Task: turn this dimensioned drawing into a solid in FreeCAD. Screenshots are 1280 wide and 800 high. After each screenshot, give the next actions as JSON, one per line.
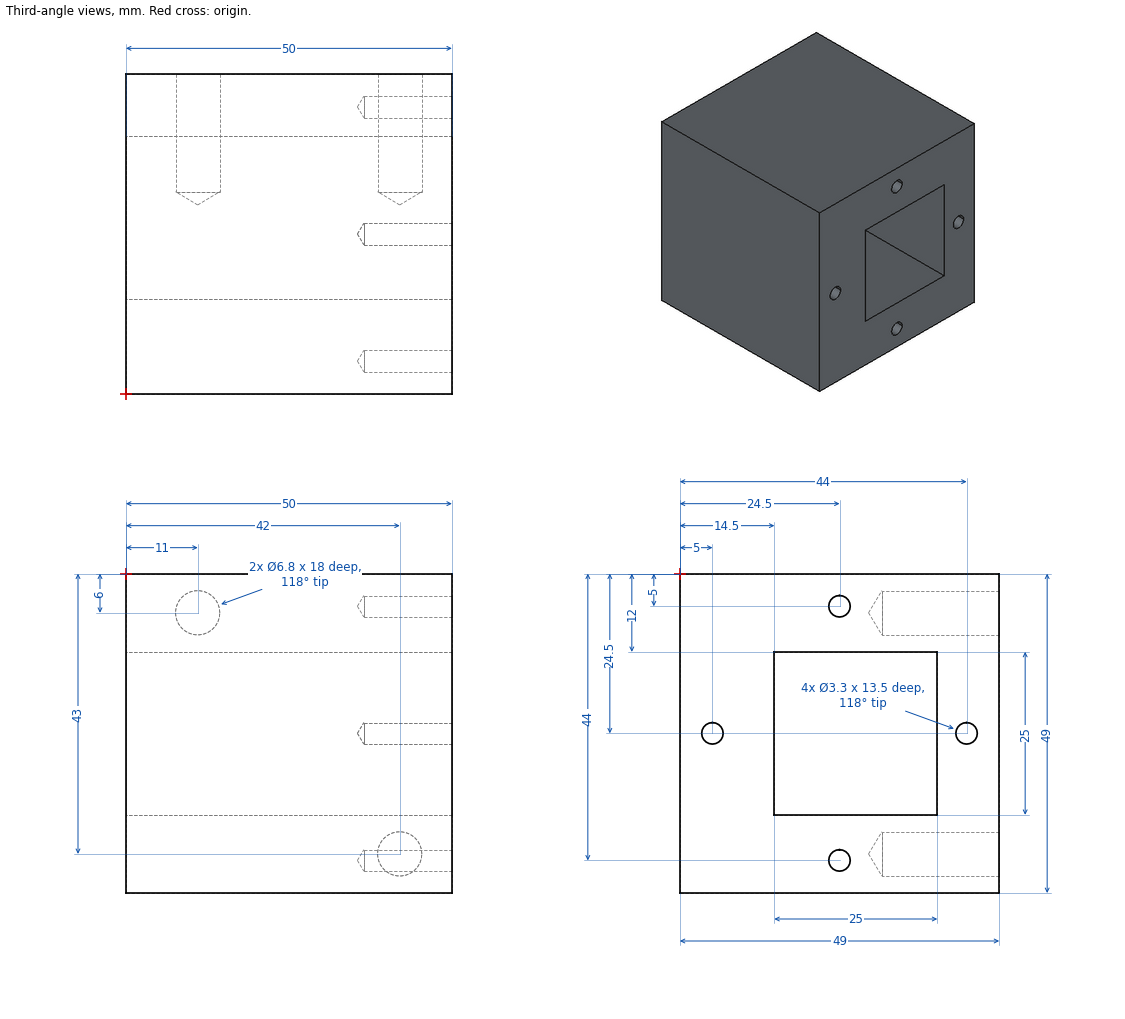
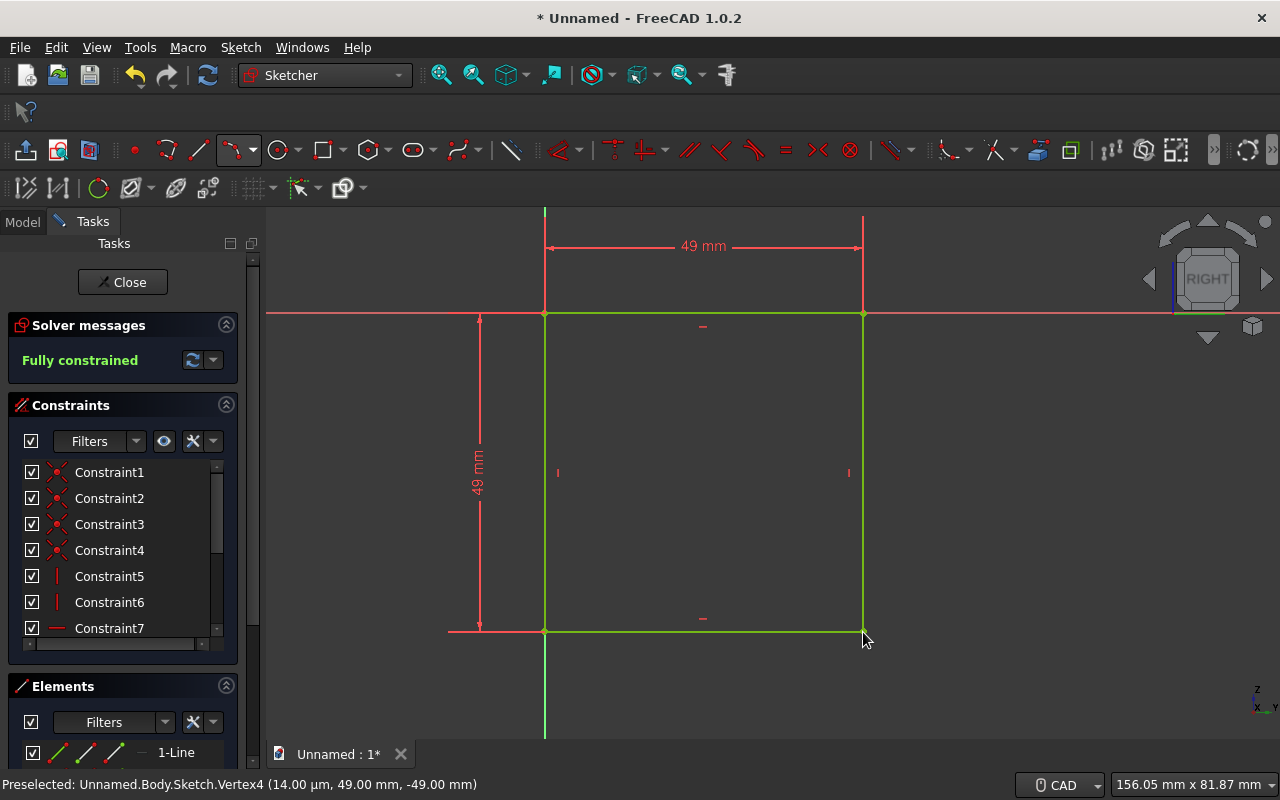
{"action": "left_click", "coordinate": [123, 282]}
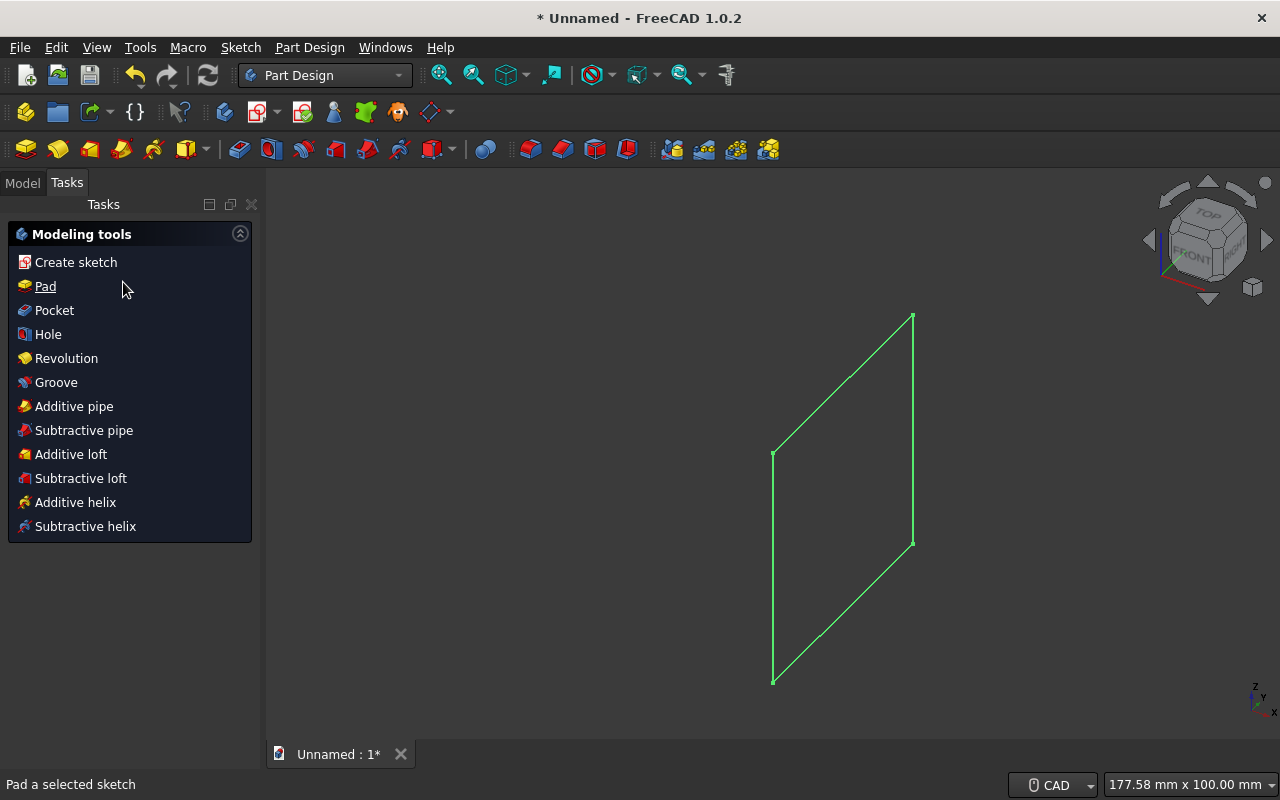
{"action": "left_click", "coordinate": [26, 150]}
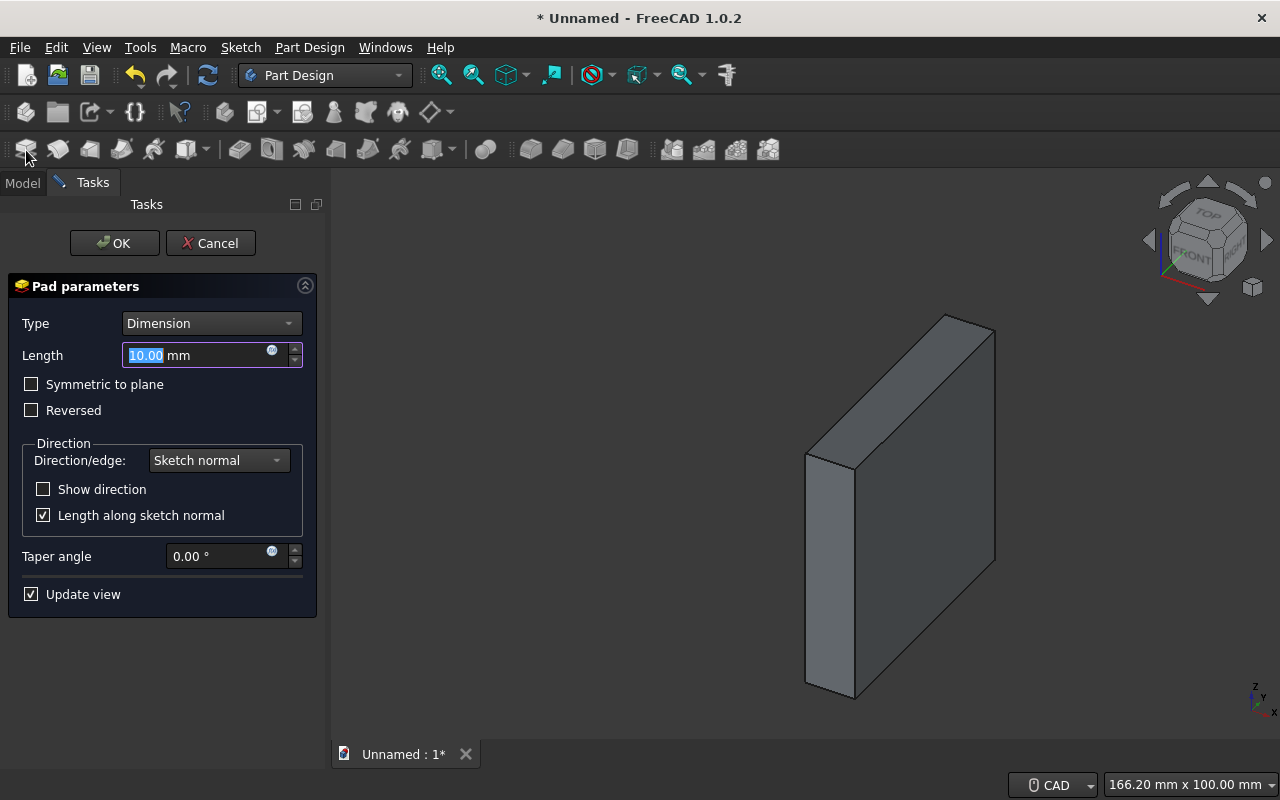
{"action": "type", "text": "50"}
{"action": "key", "text": "Tab"}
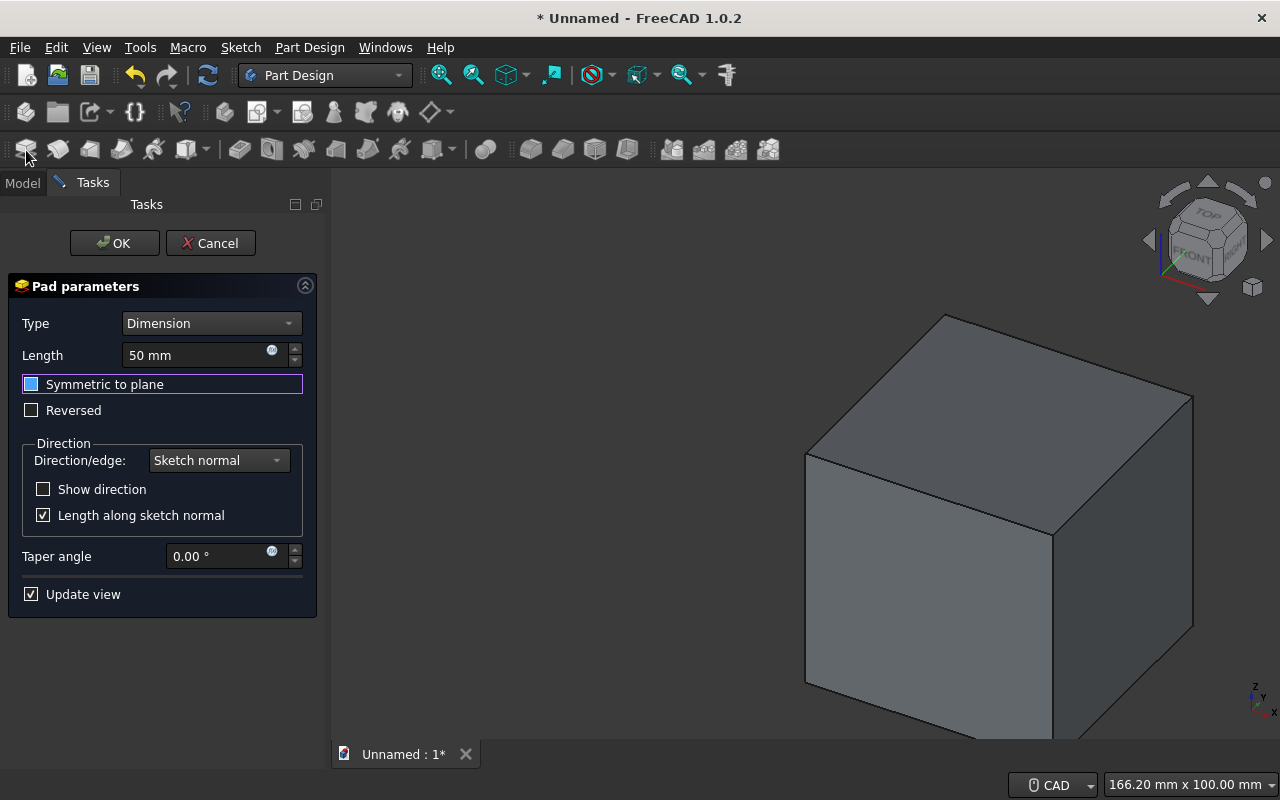
{"action": "left_click", "coordinate": [115, 243]}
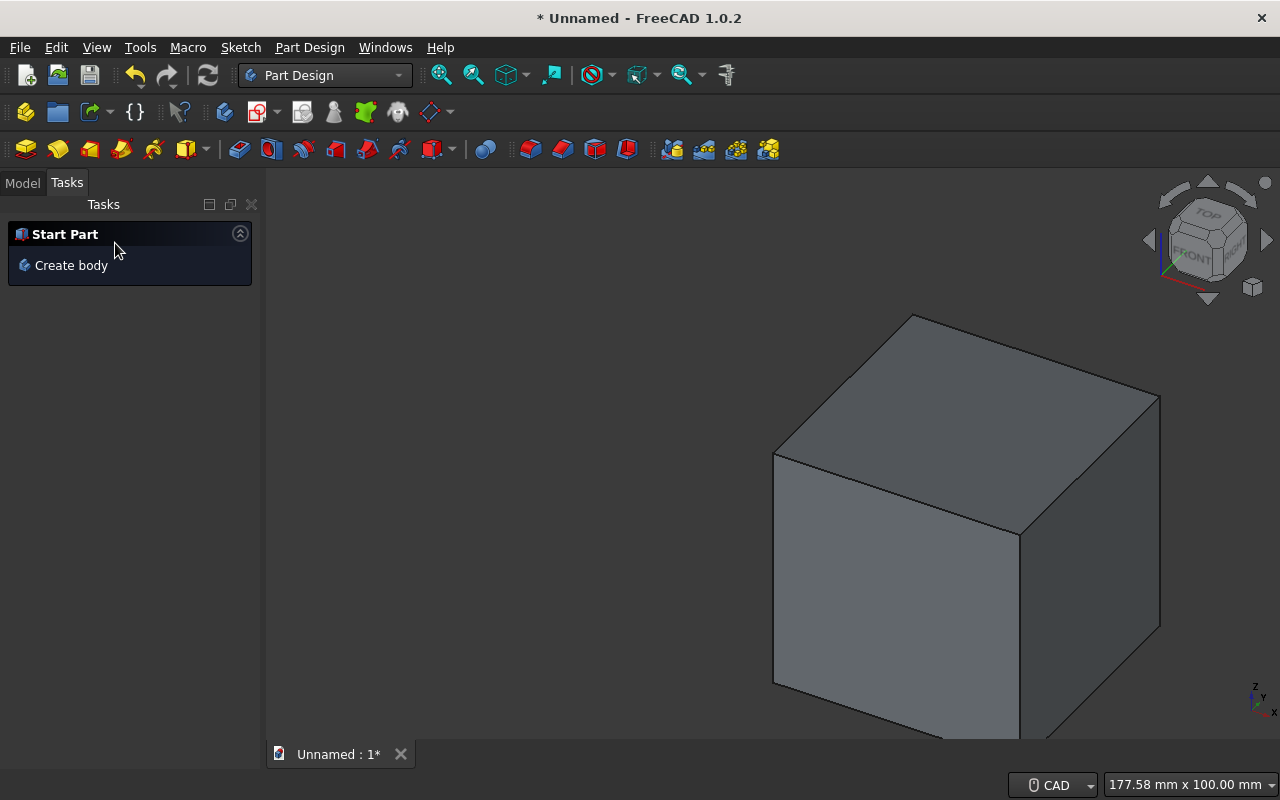
{"action": "key", "text": "v f"}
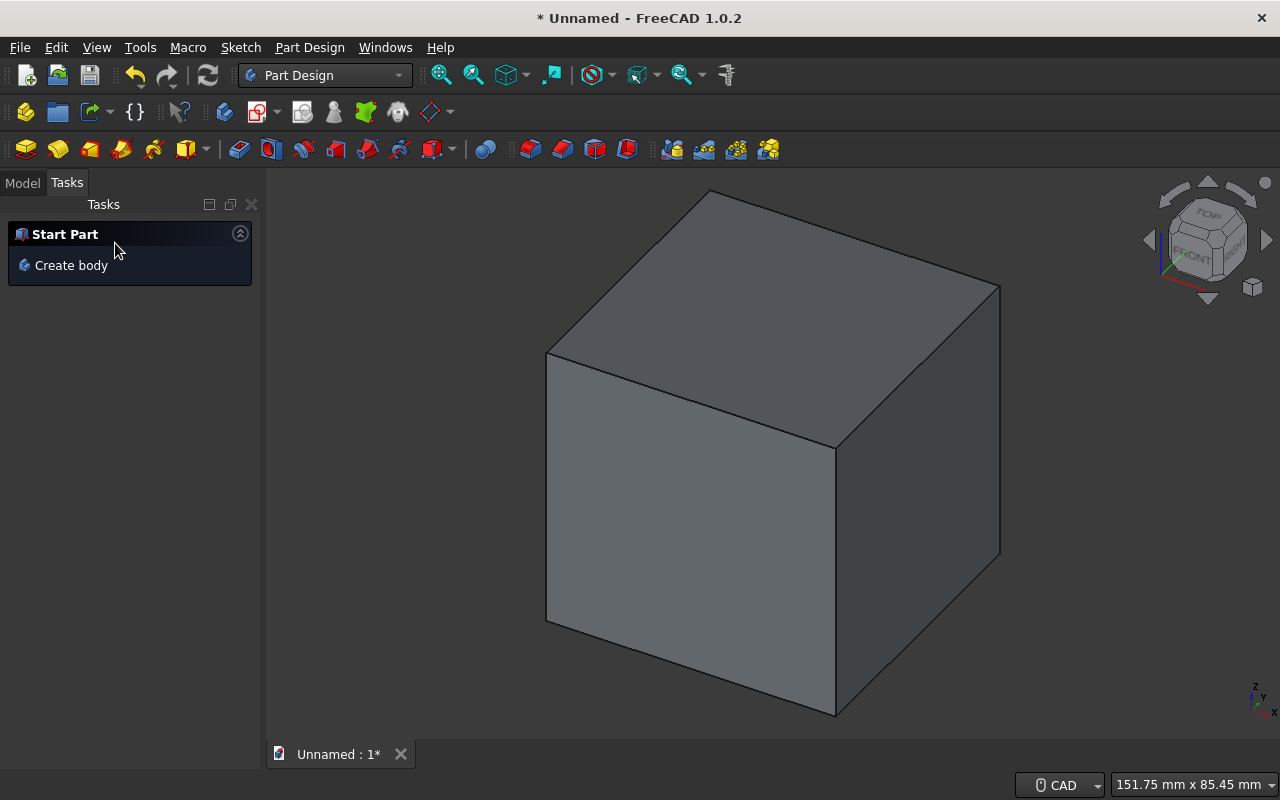
{"action": "left_click", "coordinate": [918, 500]}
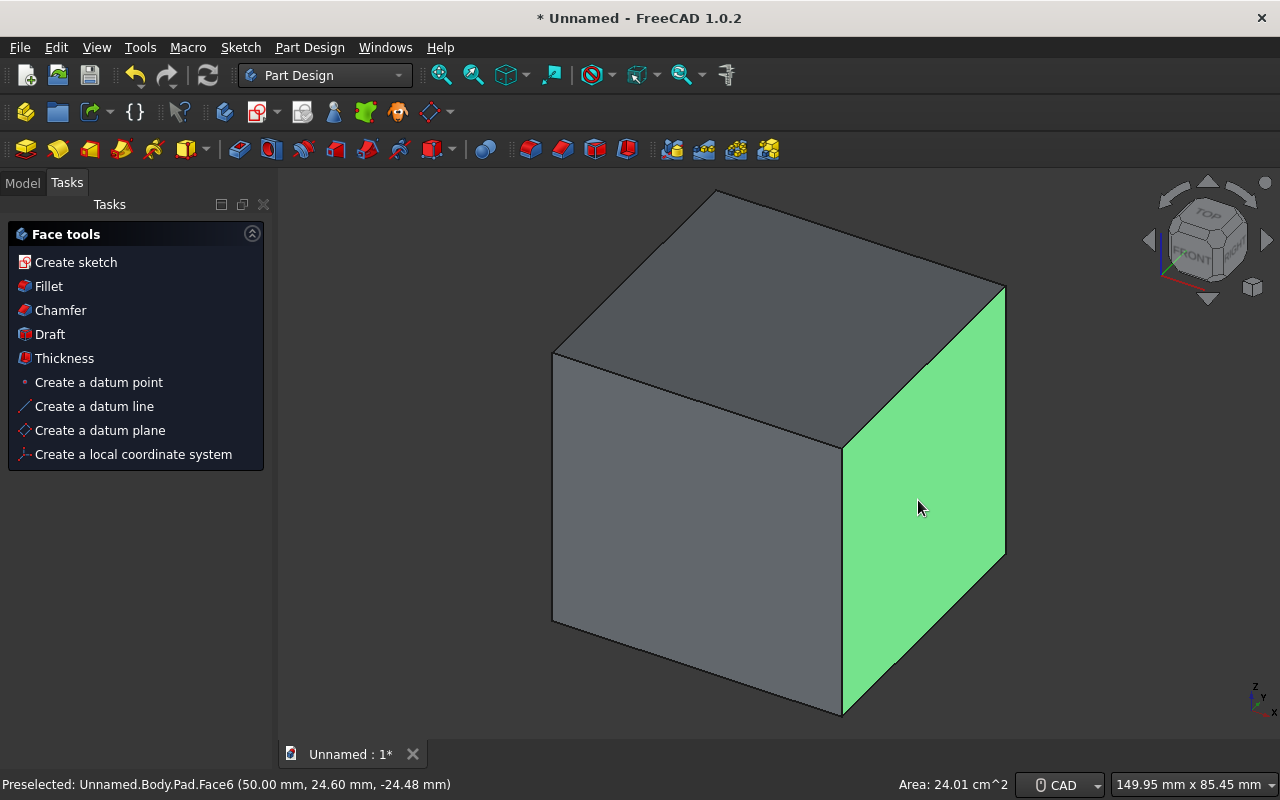
{"action": "left_click", "coordinate": [258, 112]}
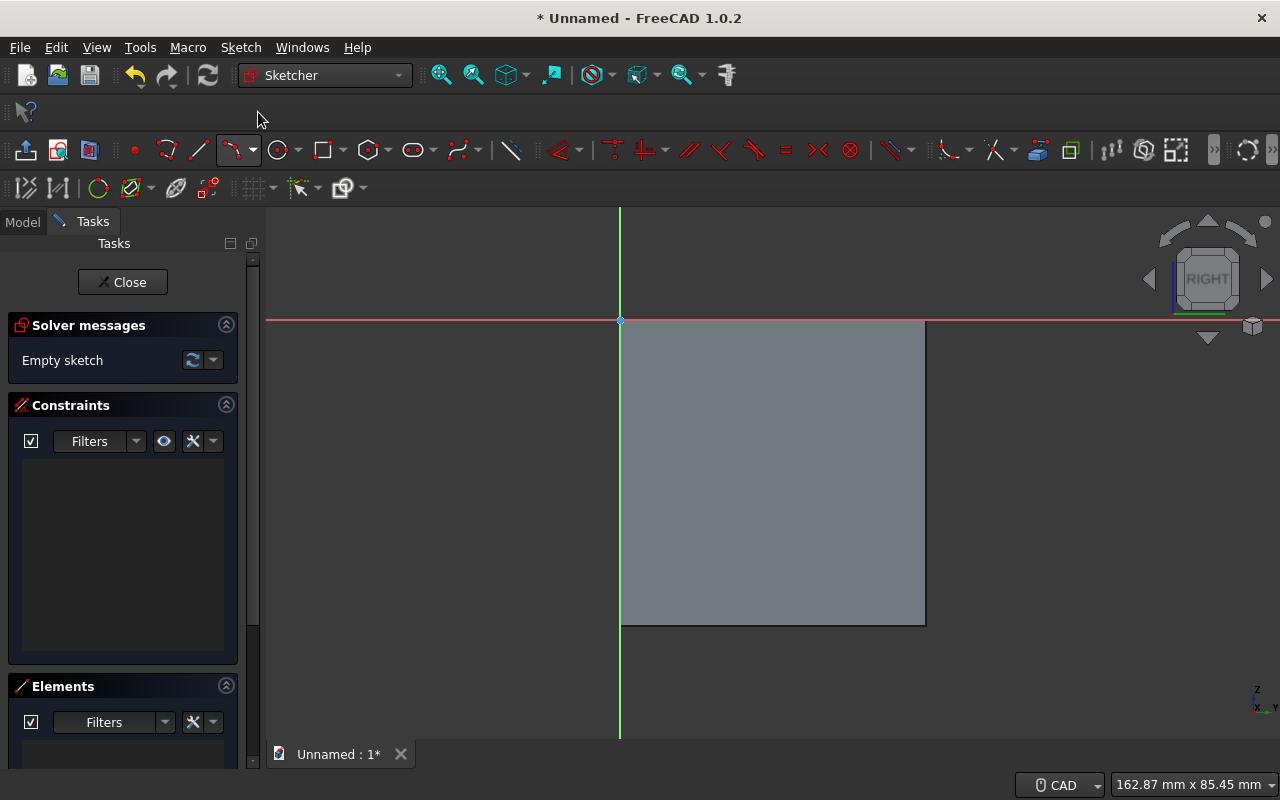
{"action": "scroll", "coordinate": [823, 360], "scroll_direction": "up", "scroll_amount": 2}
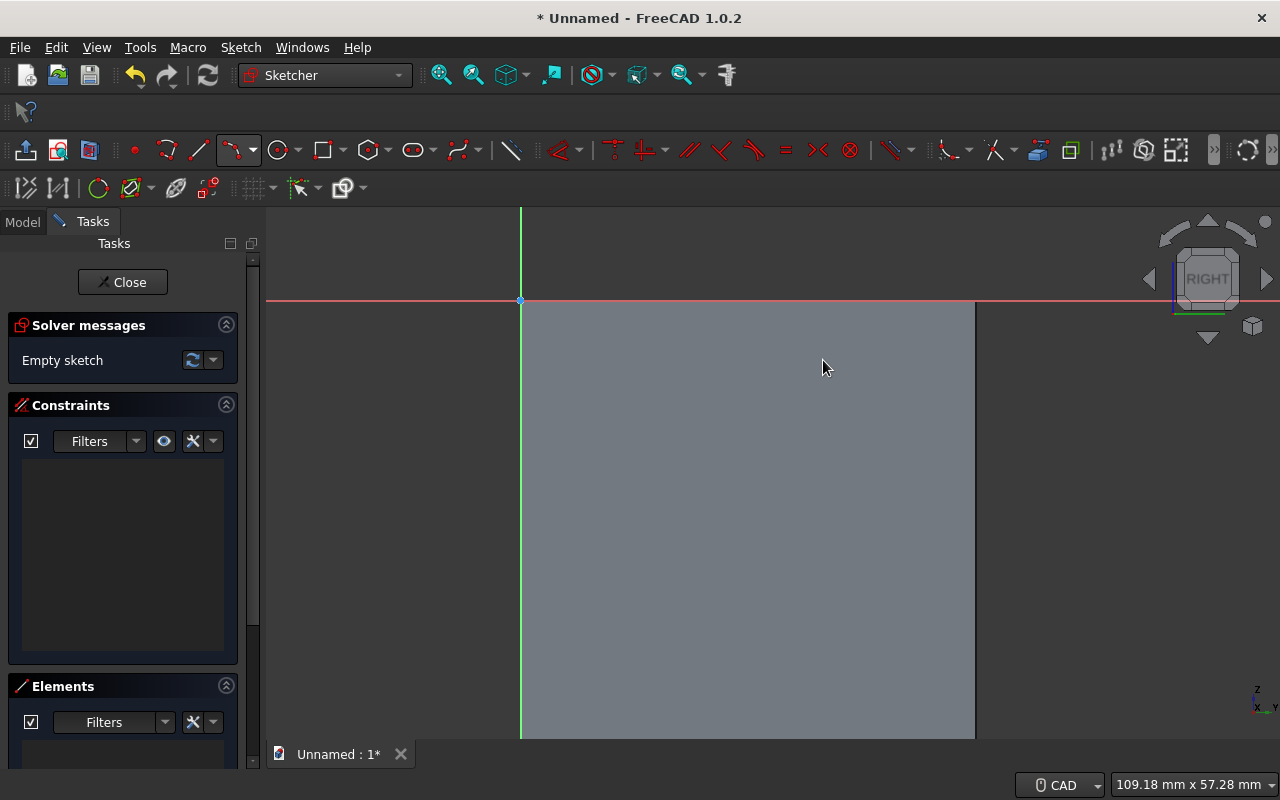
{"action": "key", "text": "g r"}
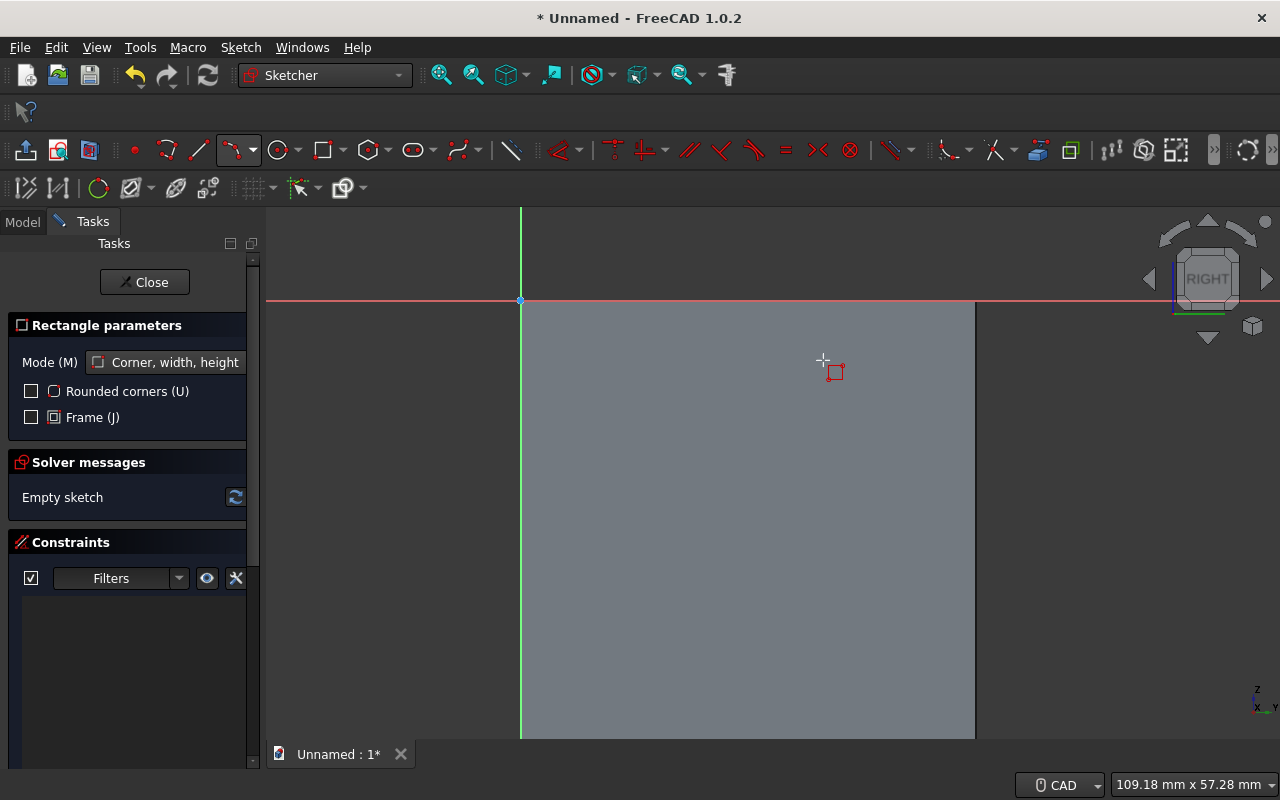
{"action": "left_click", "coordinate": [655, 412]}
{"action": "mouse_move", "coordinate": [887, 645]}